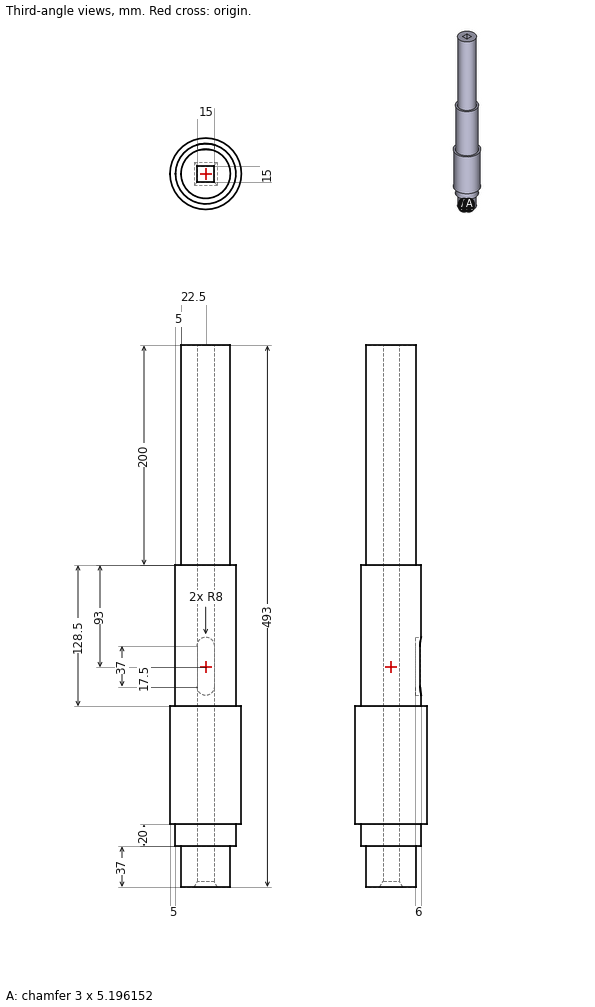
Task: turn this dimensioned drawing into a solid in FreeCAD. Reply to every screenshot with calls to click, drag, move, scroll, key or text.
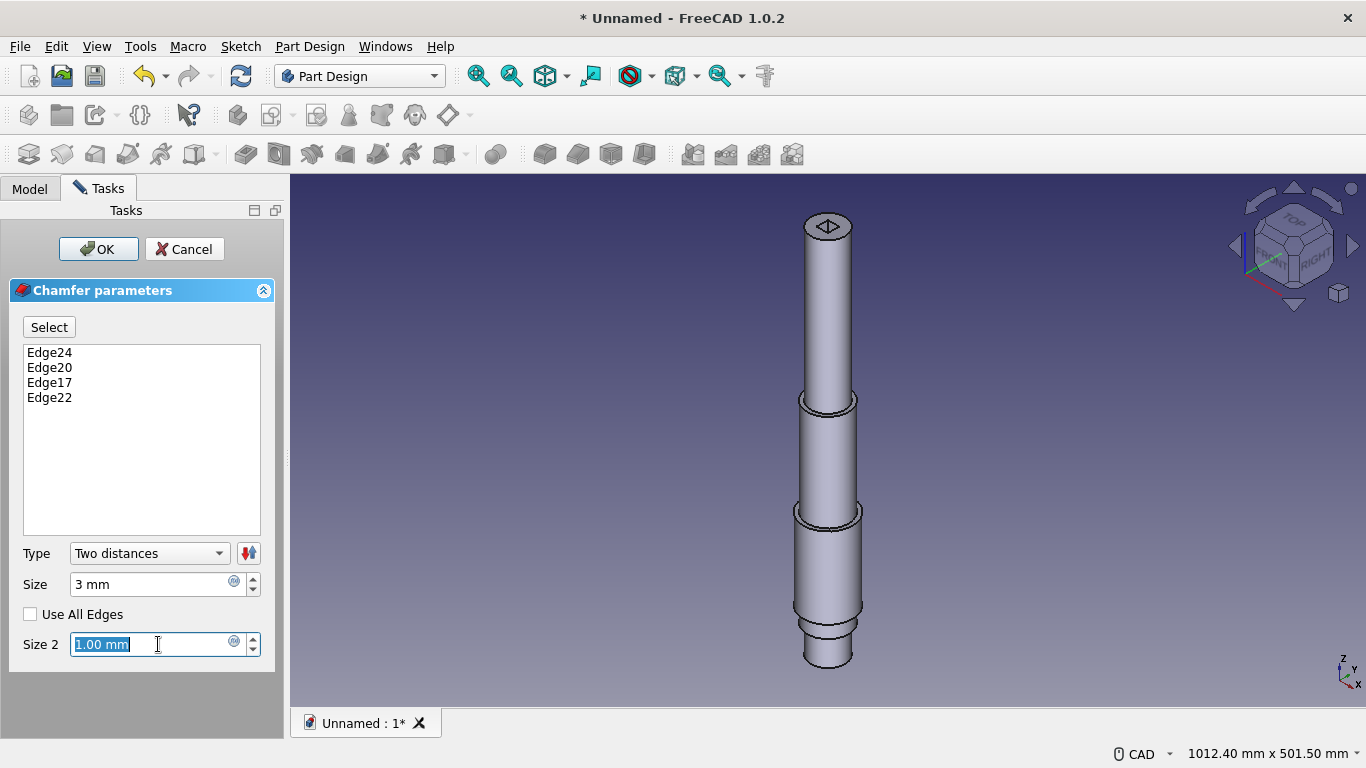
text(5.196152)
key(Tab)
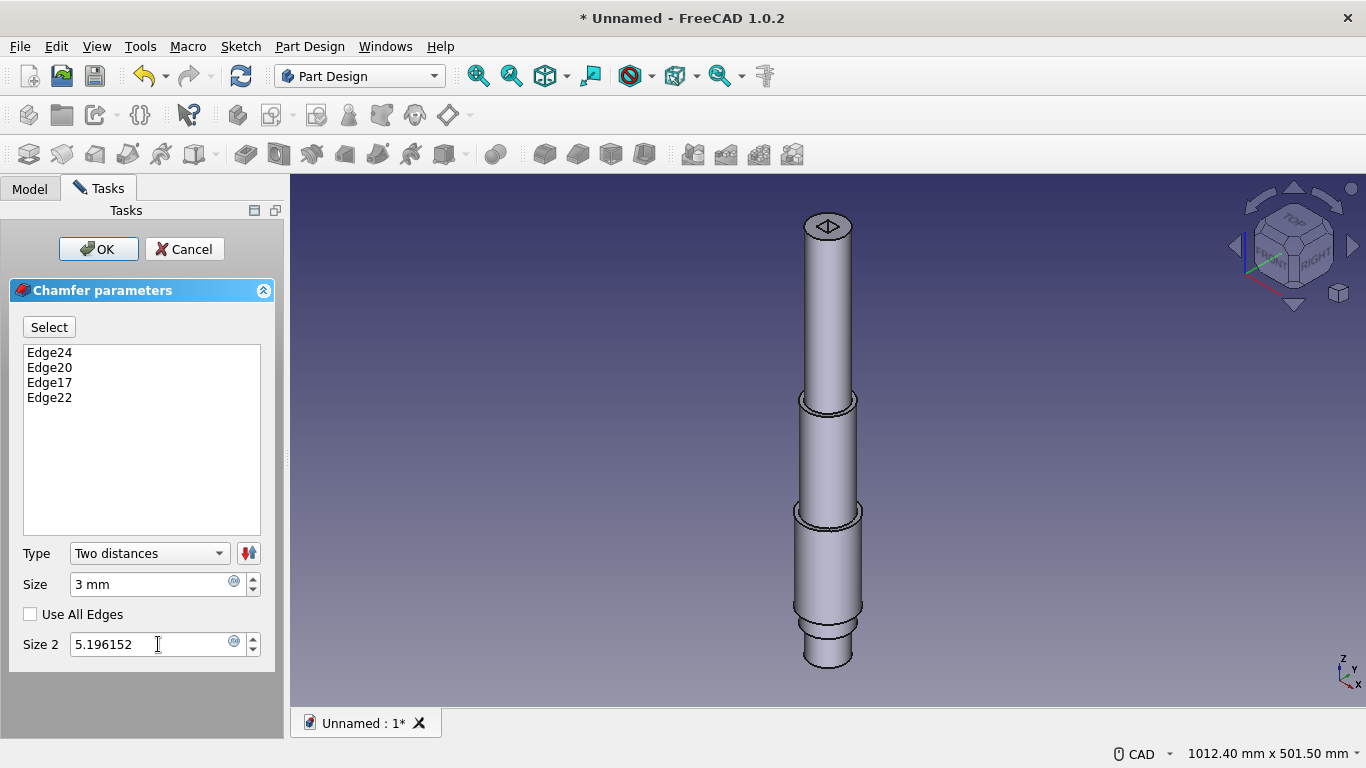
click(249, 554)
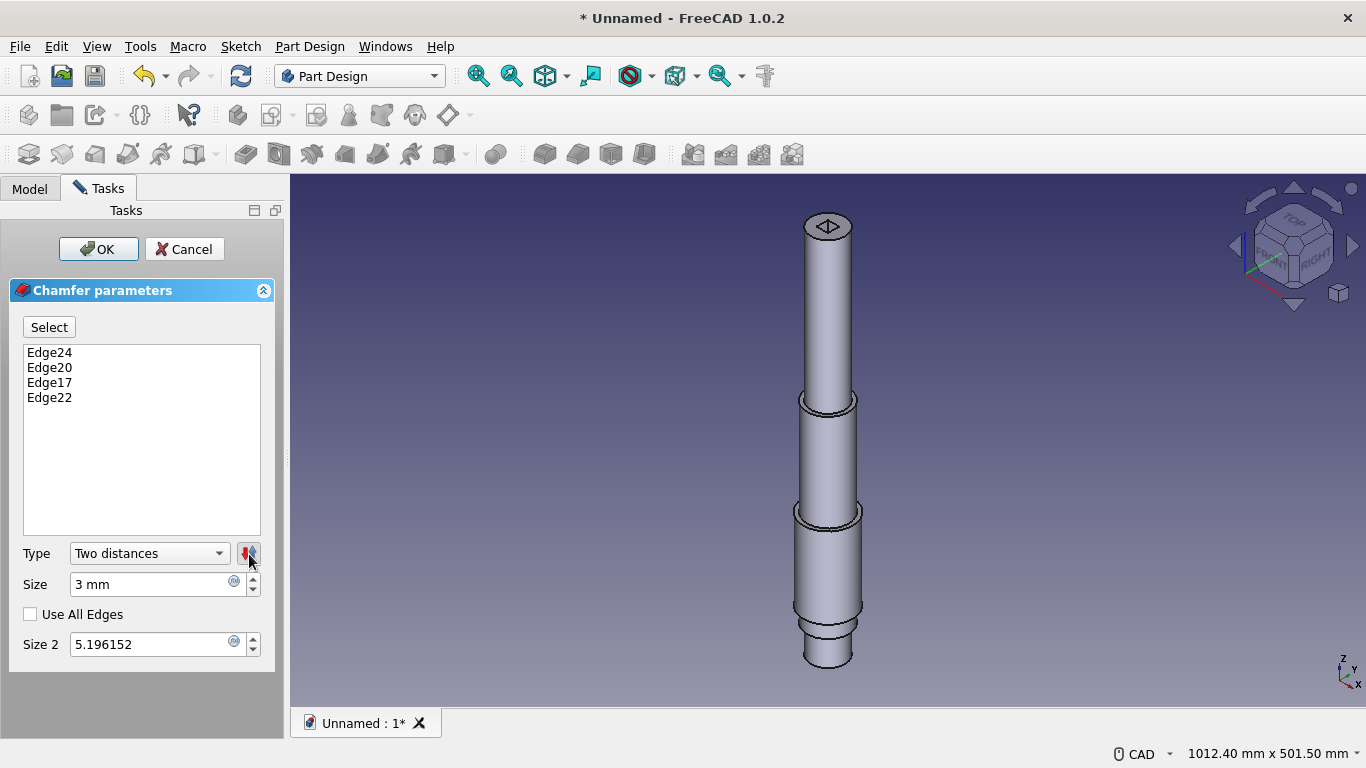
click(99, 249)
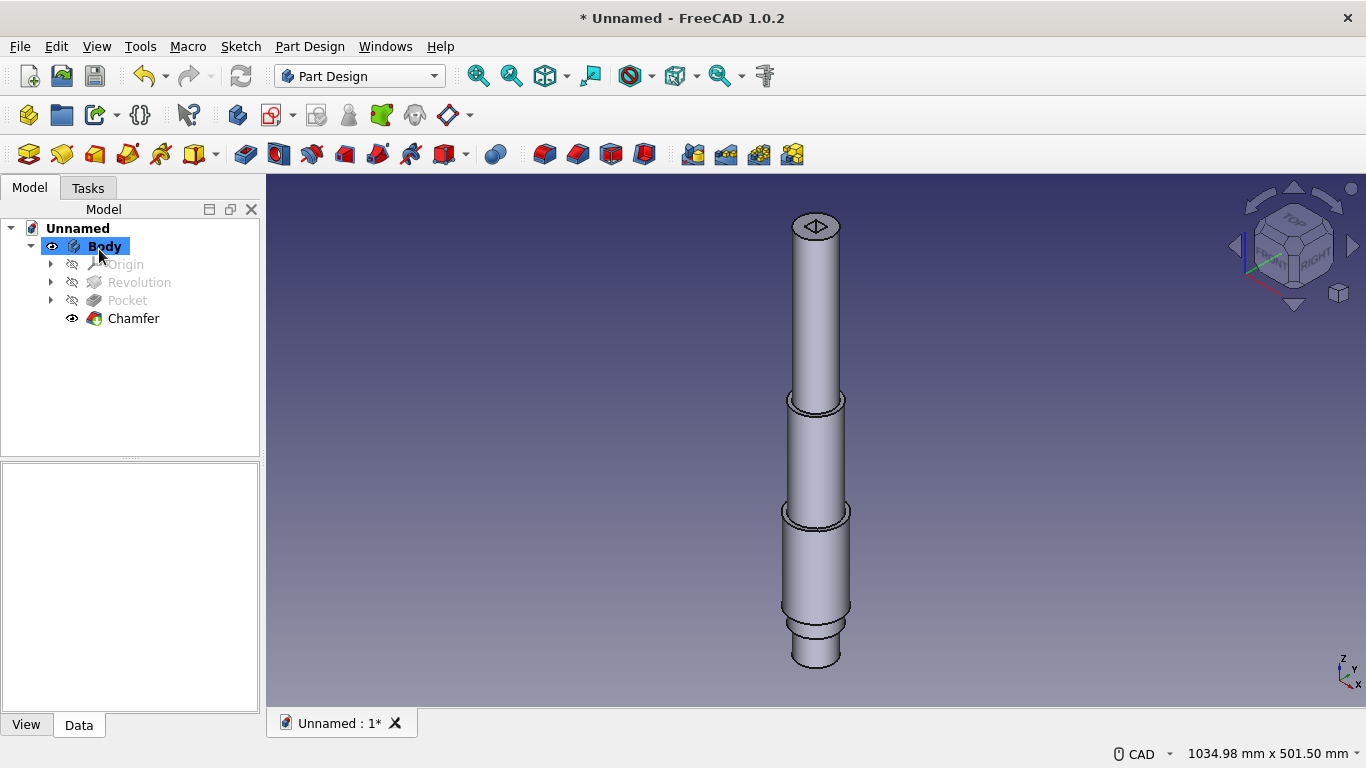
click(51, 264)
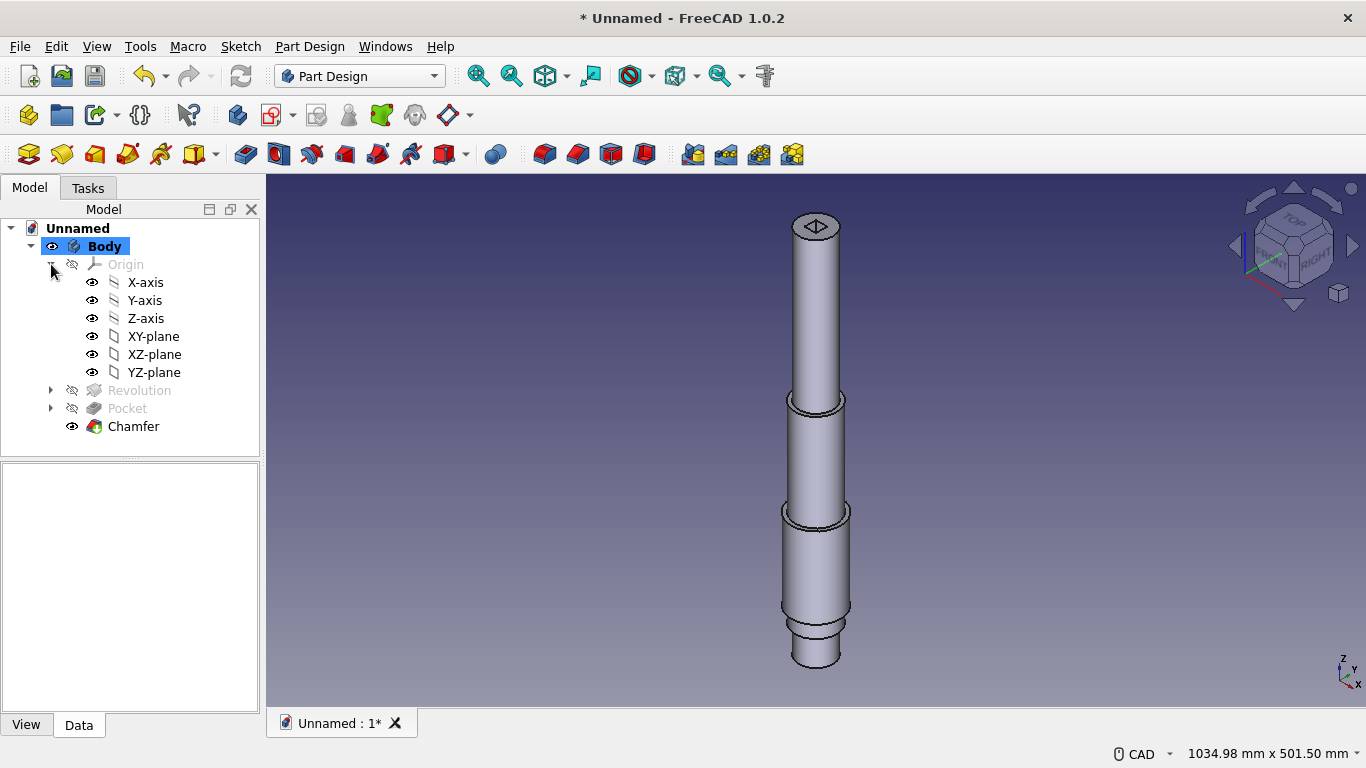
click(137, 354)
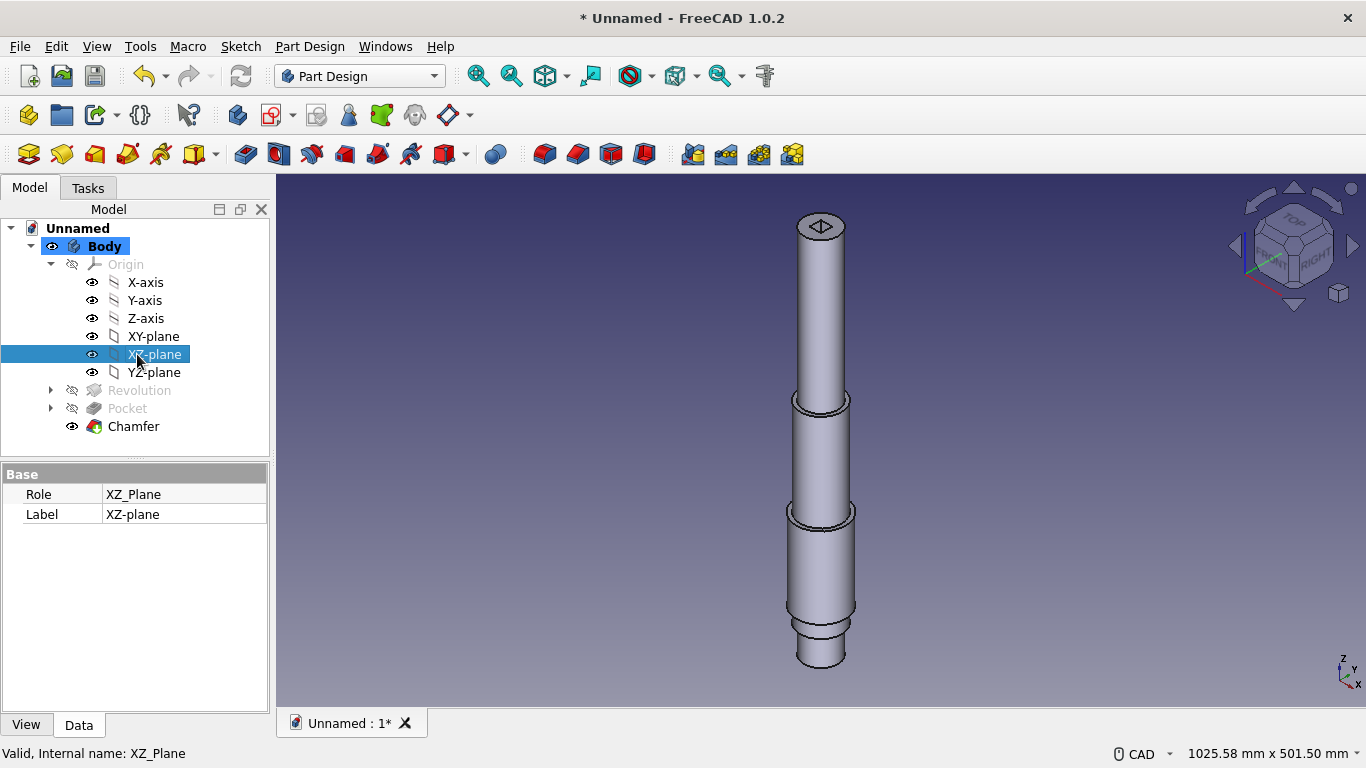
click(448, 116)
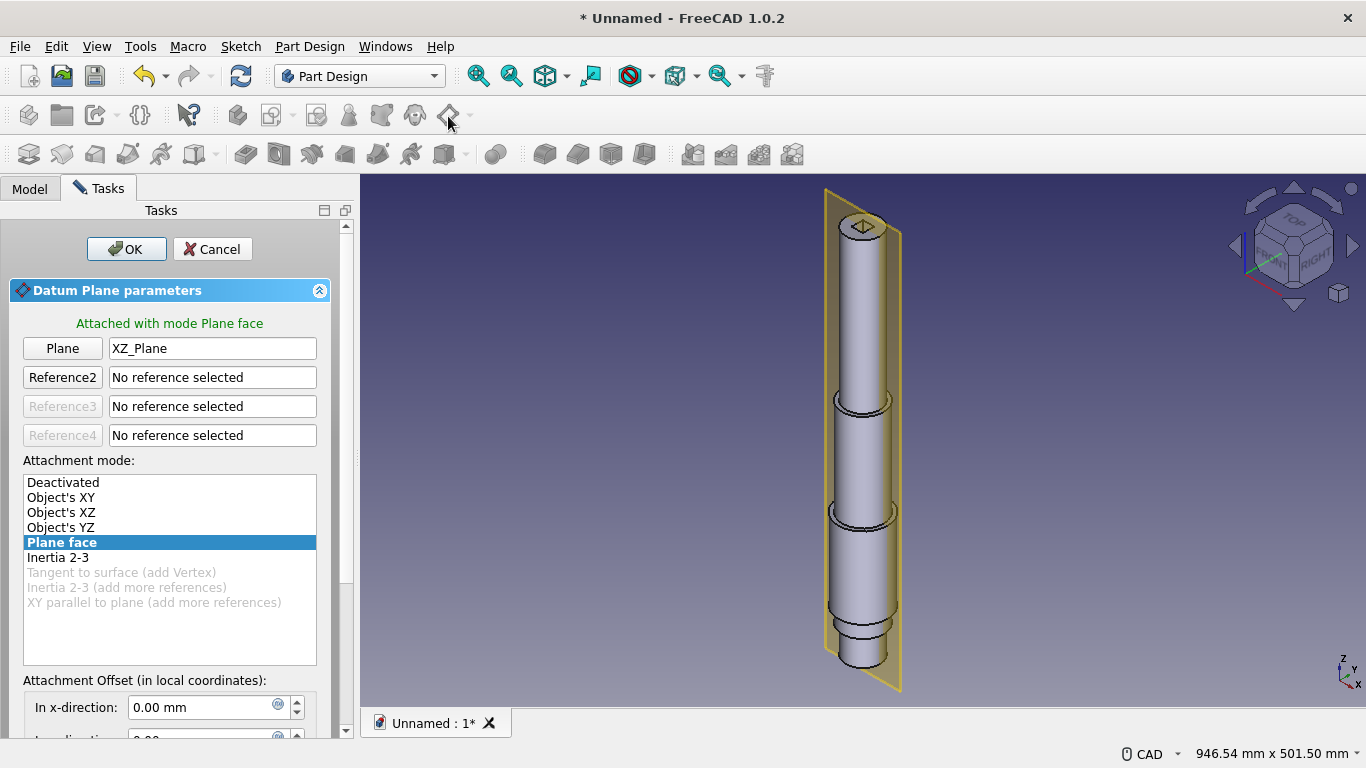
scroll(346, 479, down, 2)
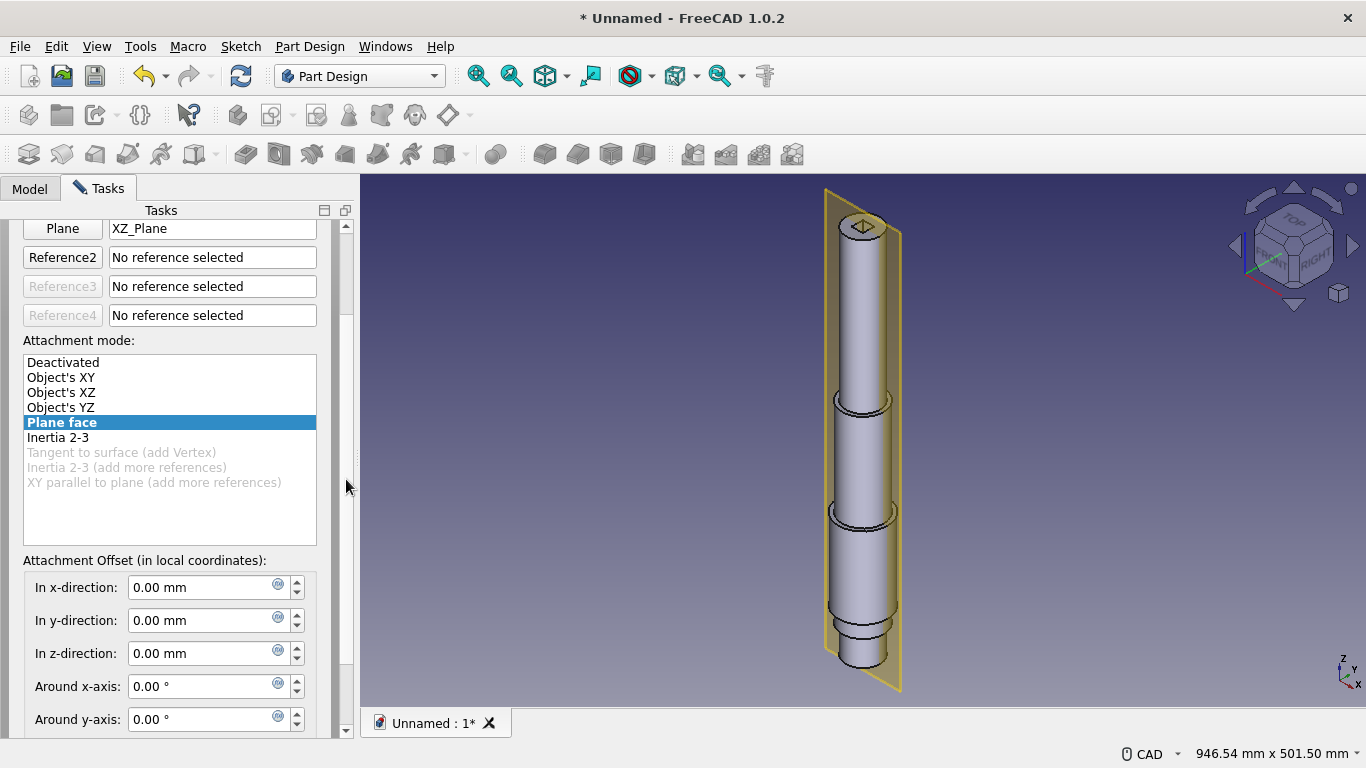
triple_click(210, 654)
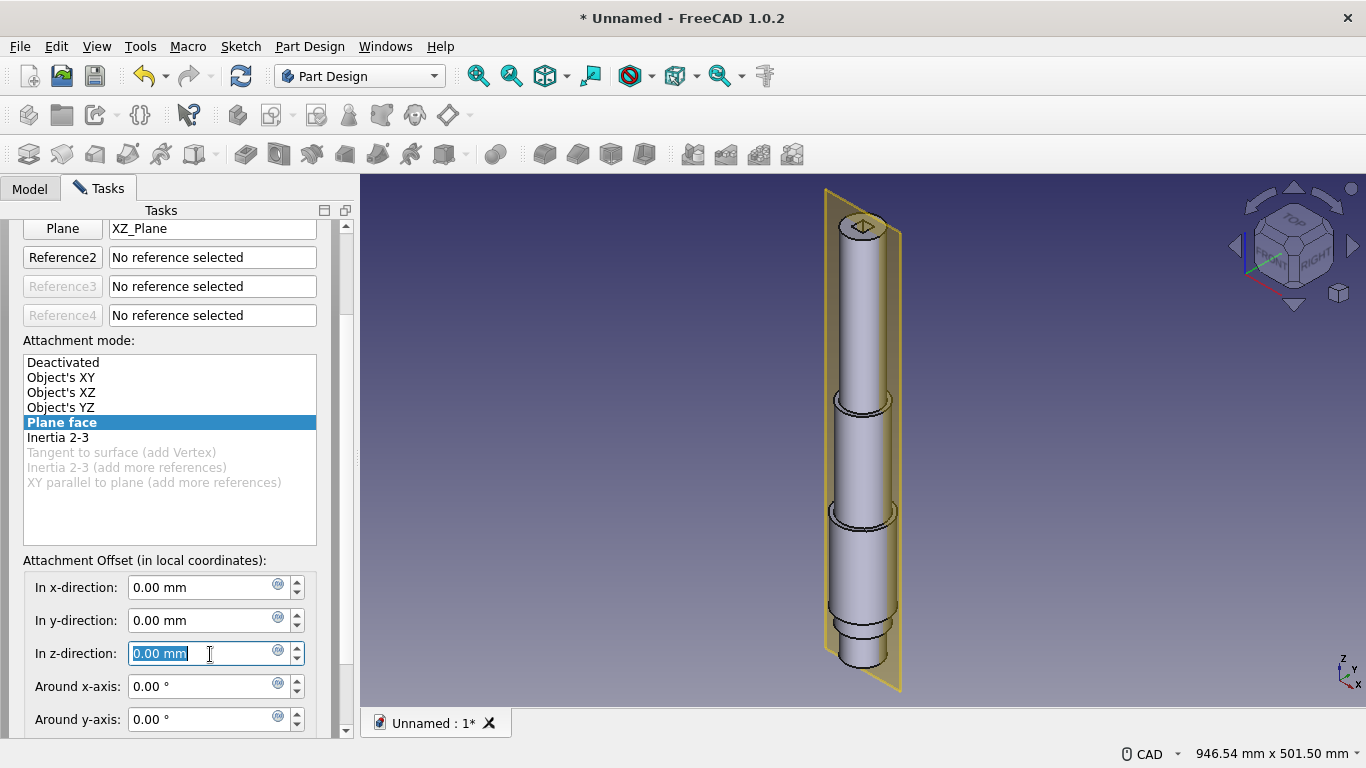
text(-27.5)
key(Tab)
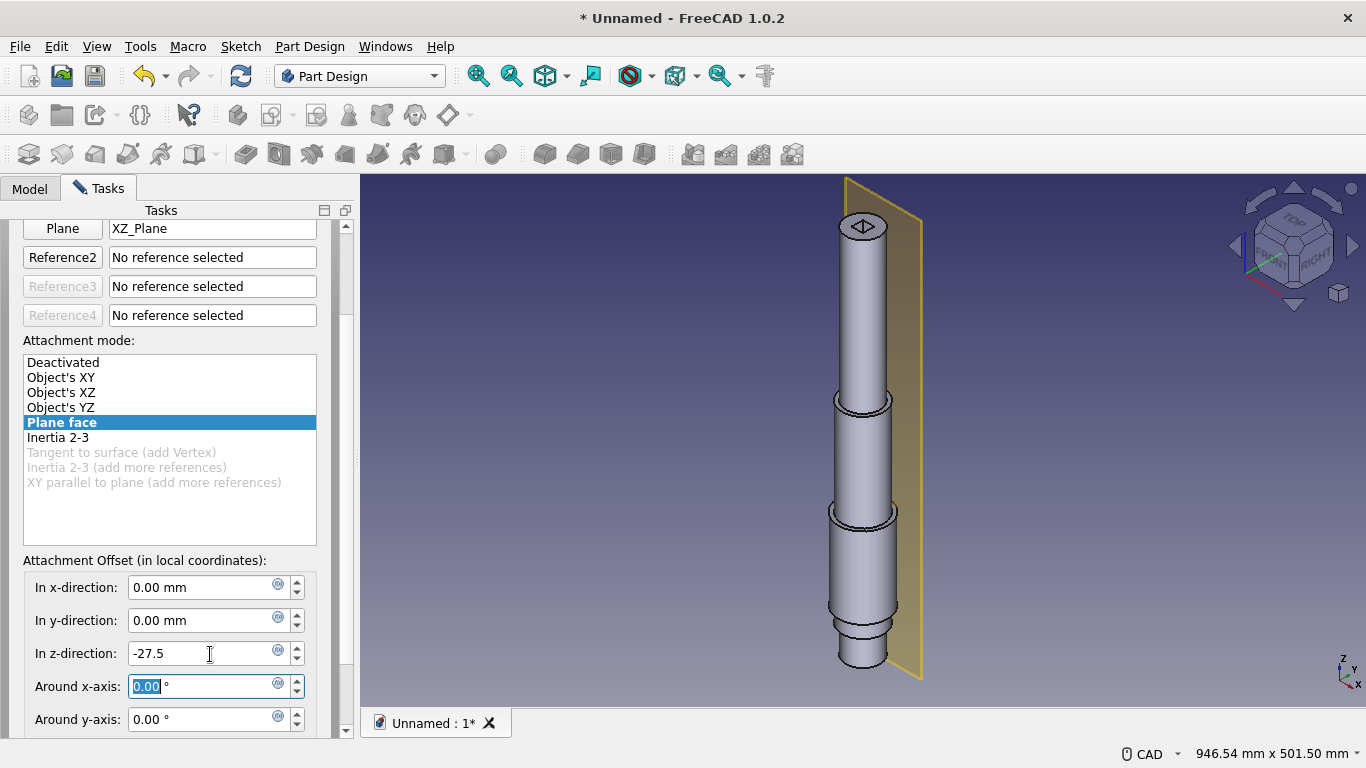
scroll(346, 479, up, 3)